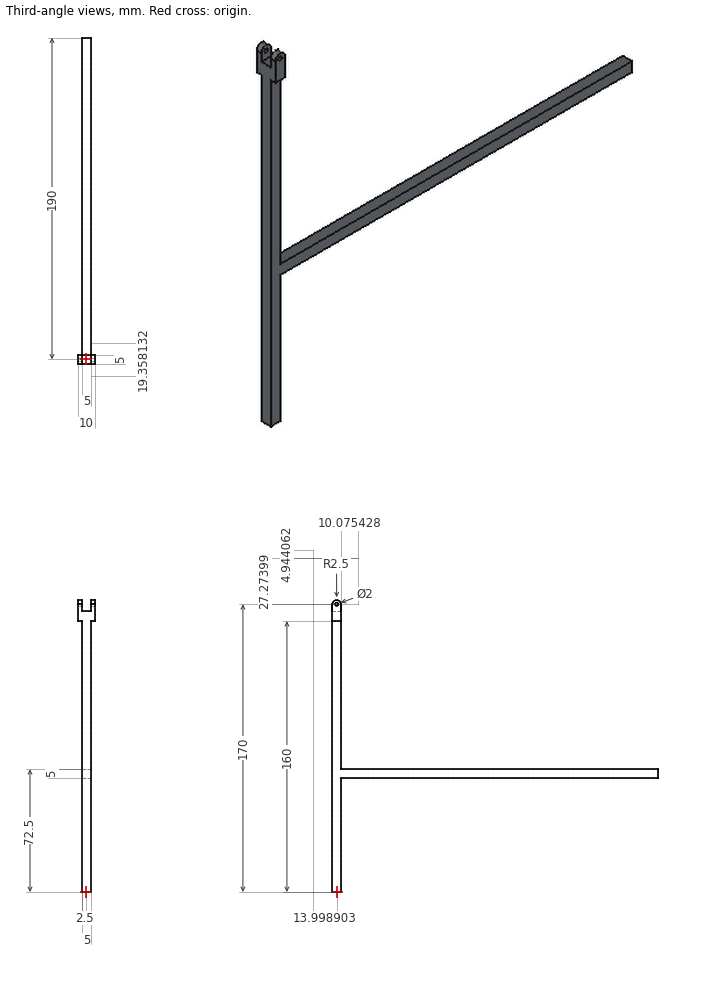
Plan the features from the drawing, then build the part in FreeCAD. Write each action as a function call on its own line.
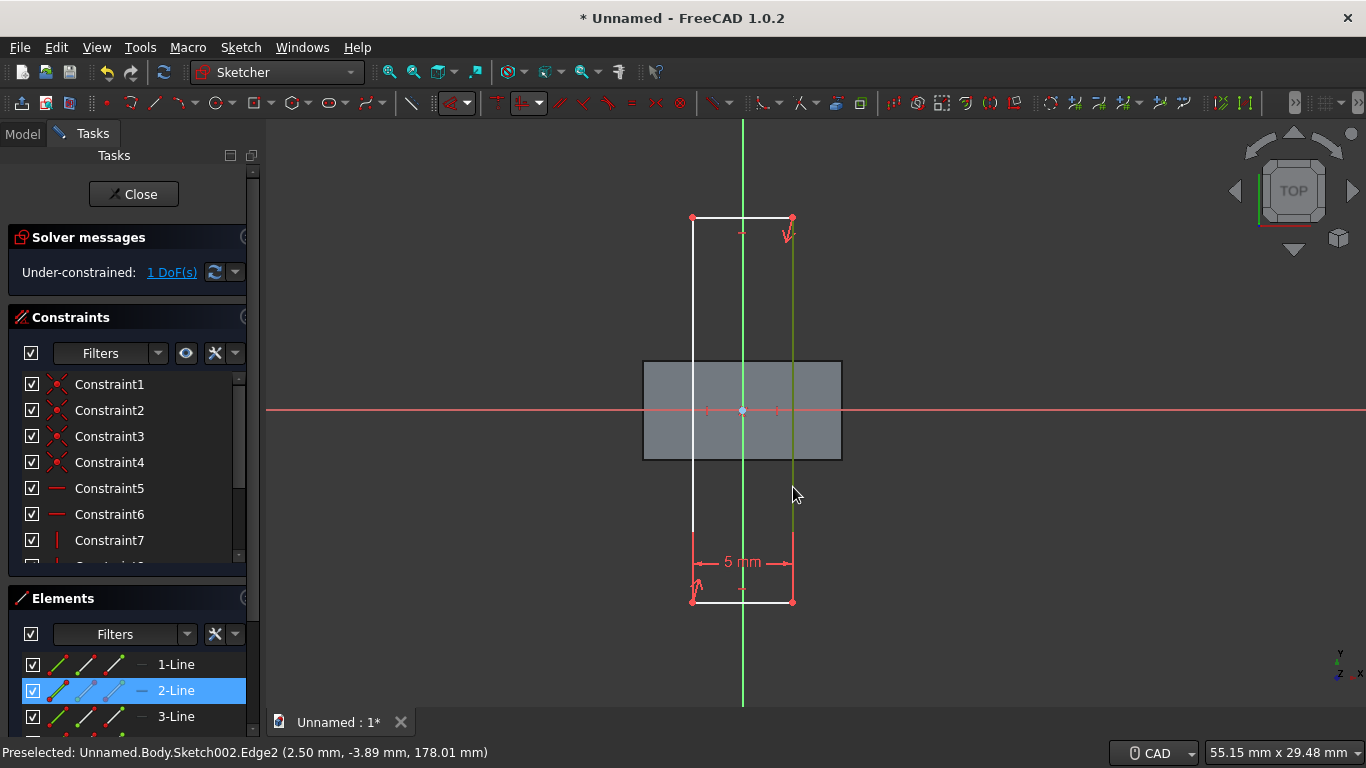
click(470, 104)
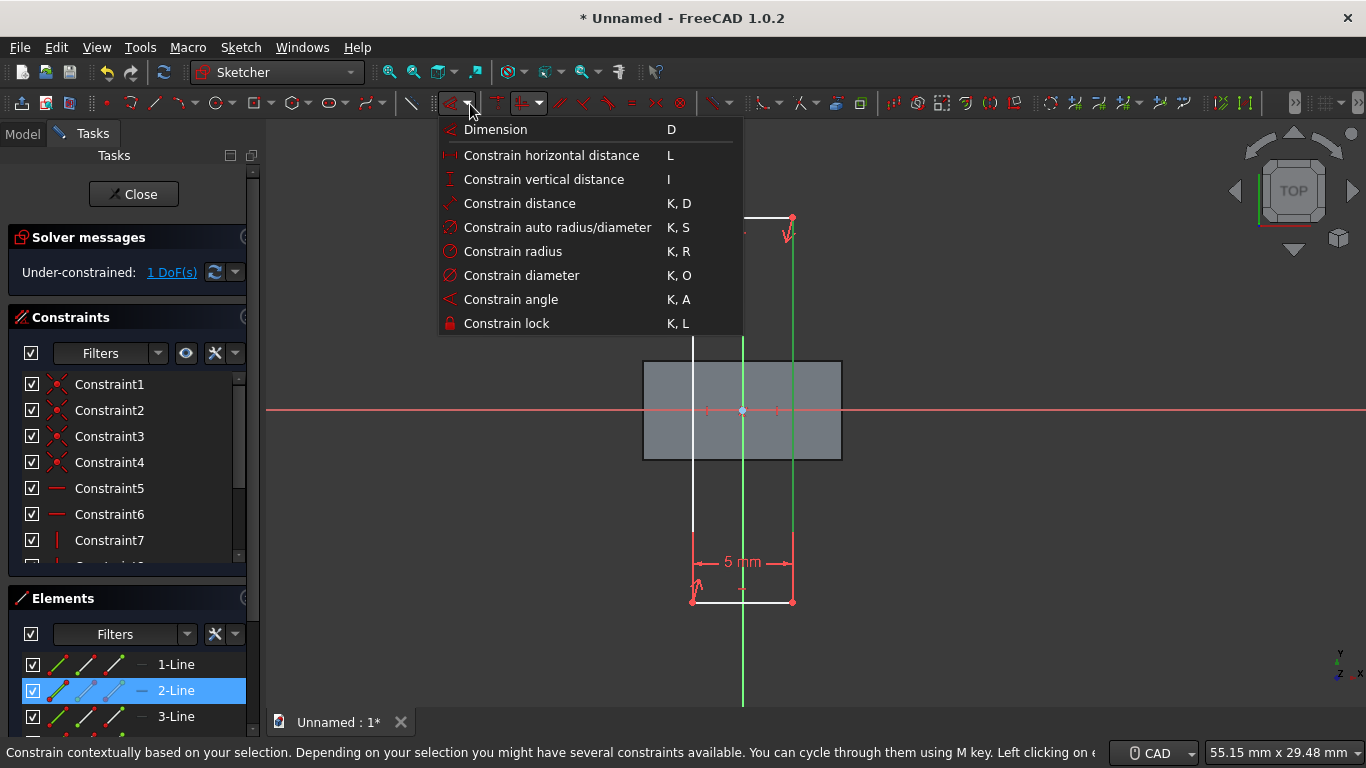
click(591, 179)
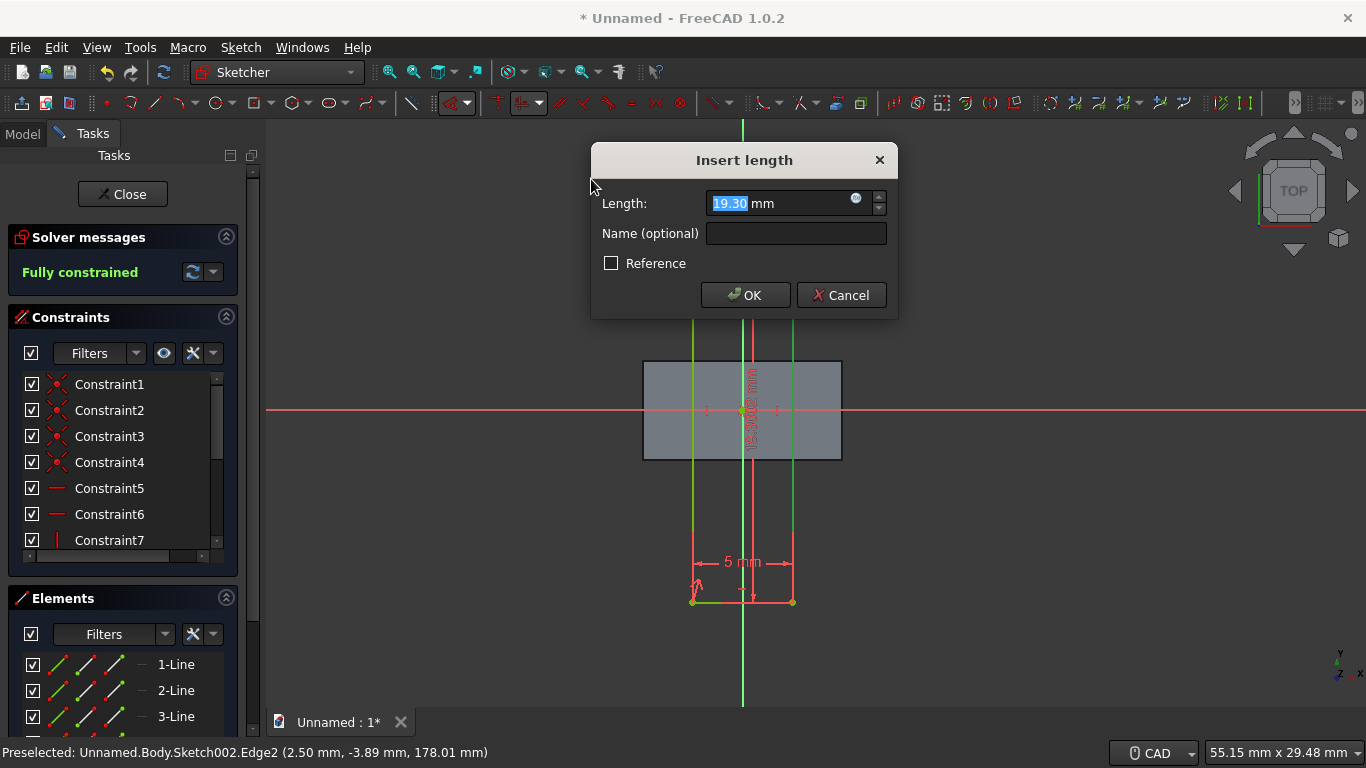
text(19.358132)
key(Return)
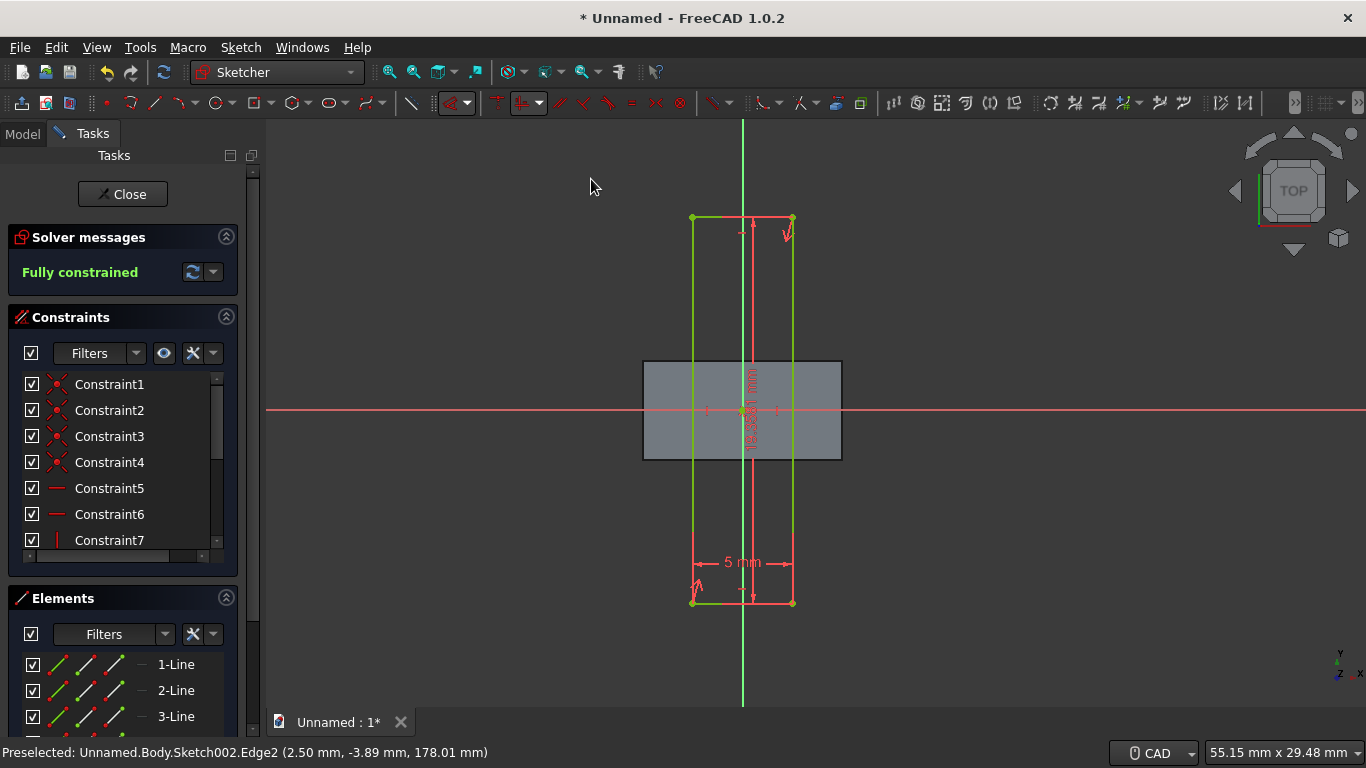
click(123, 194)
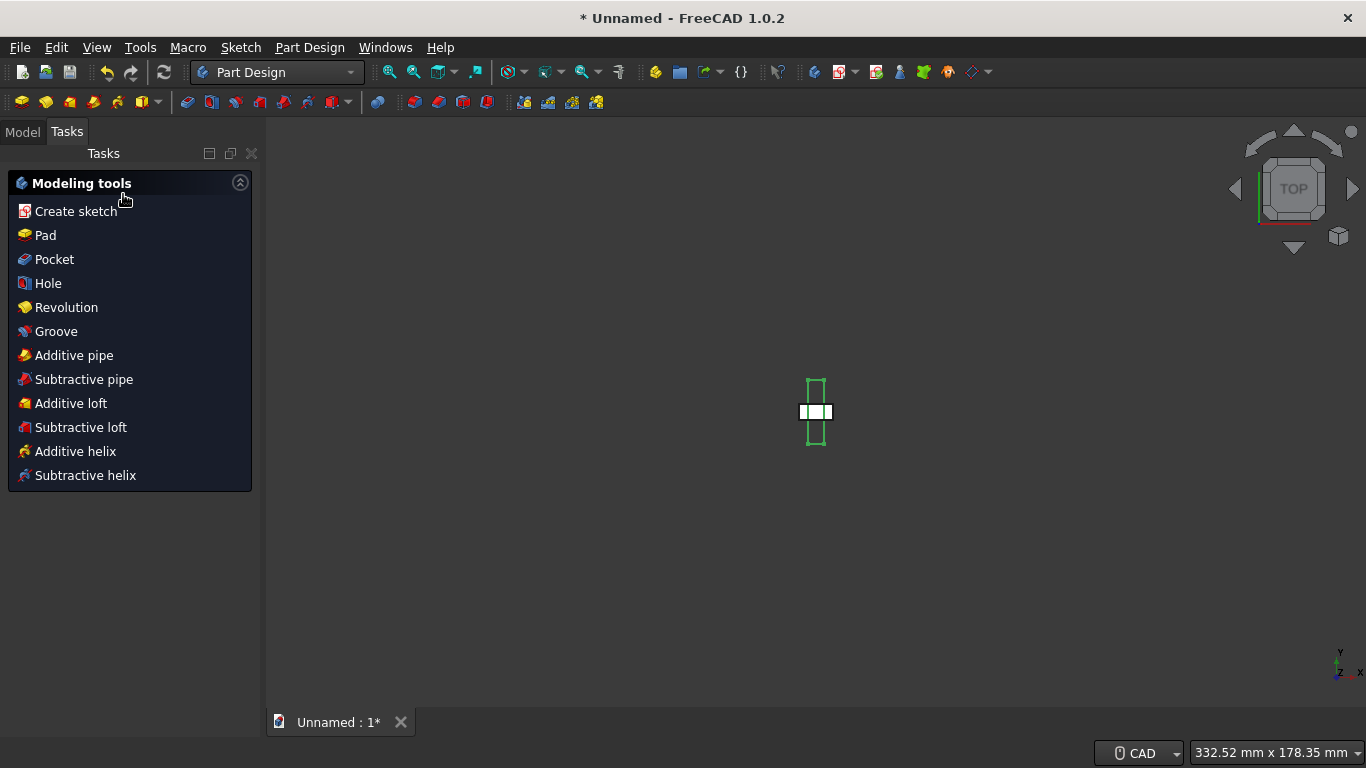
click(188, 102)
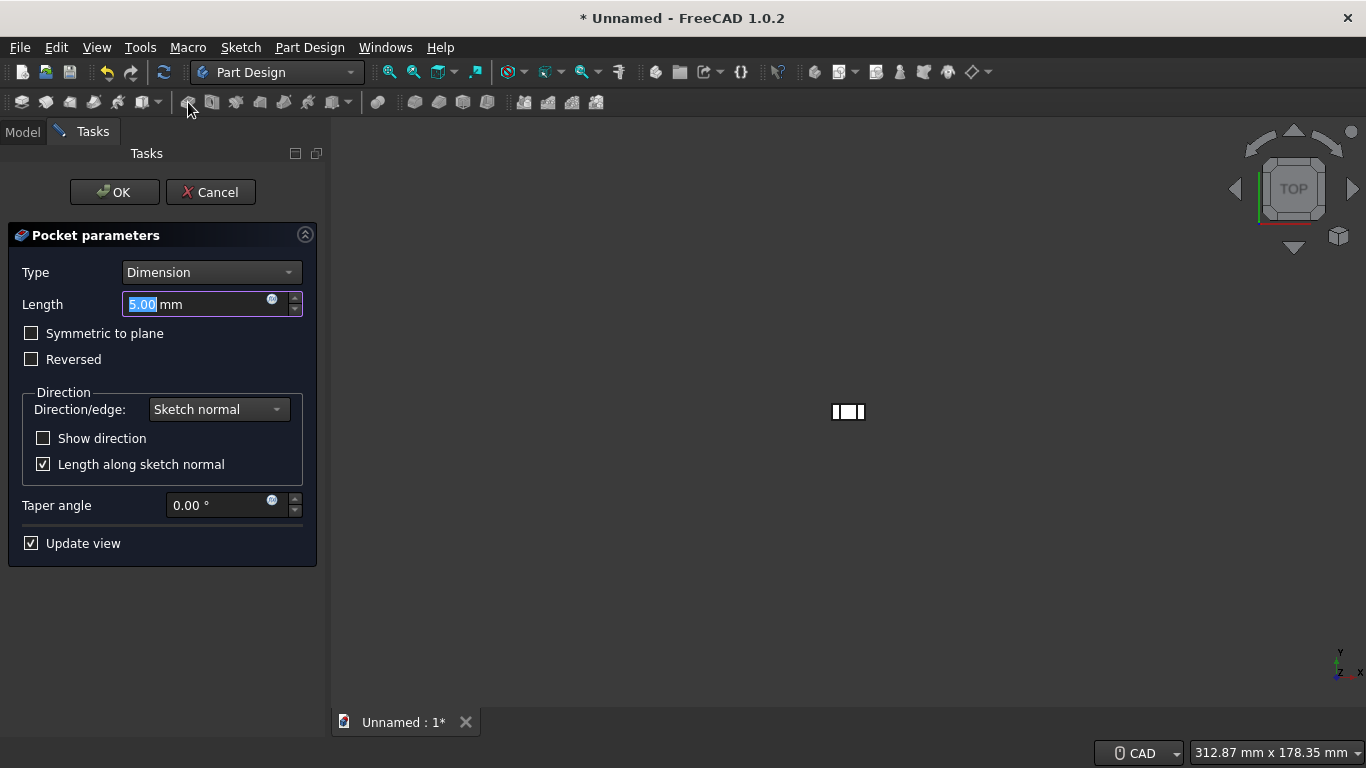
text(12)
key(Tab)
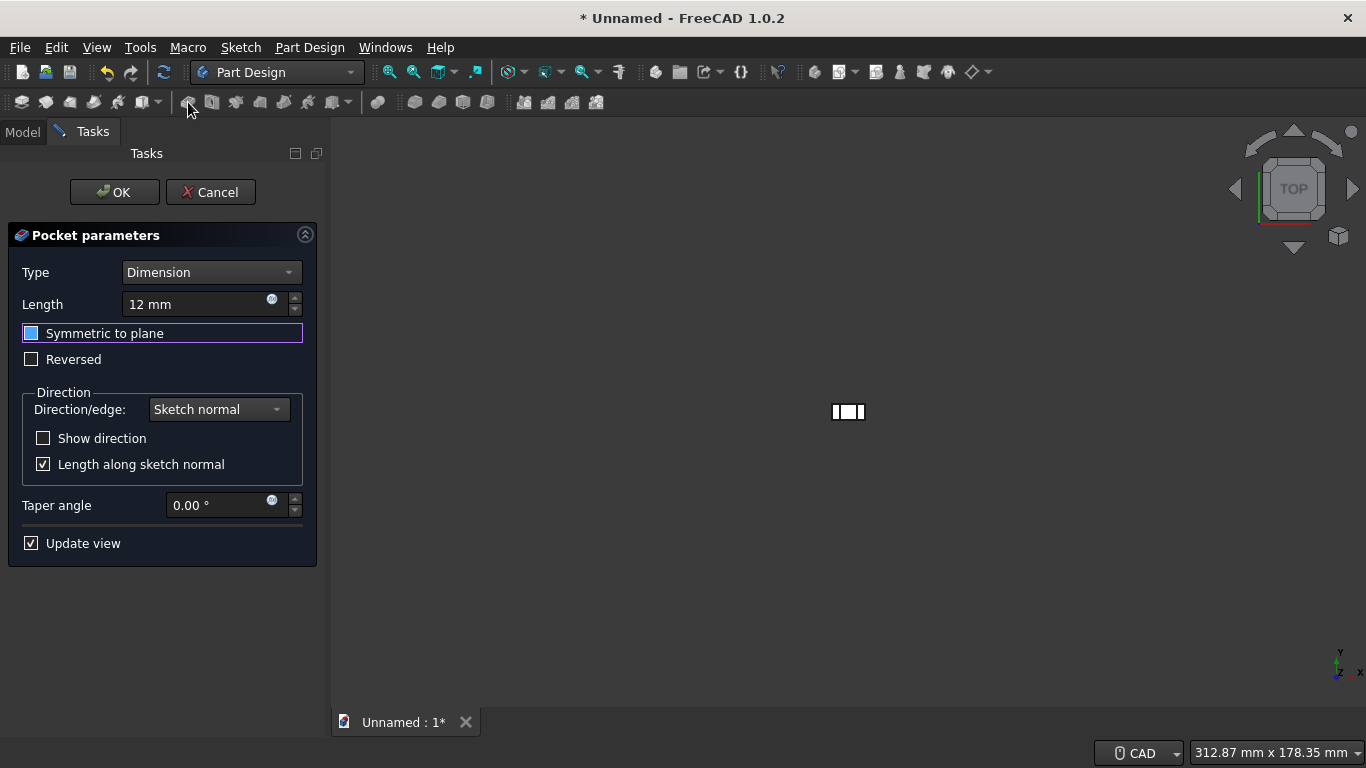
click(115, 192)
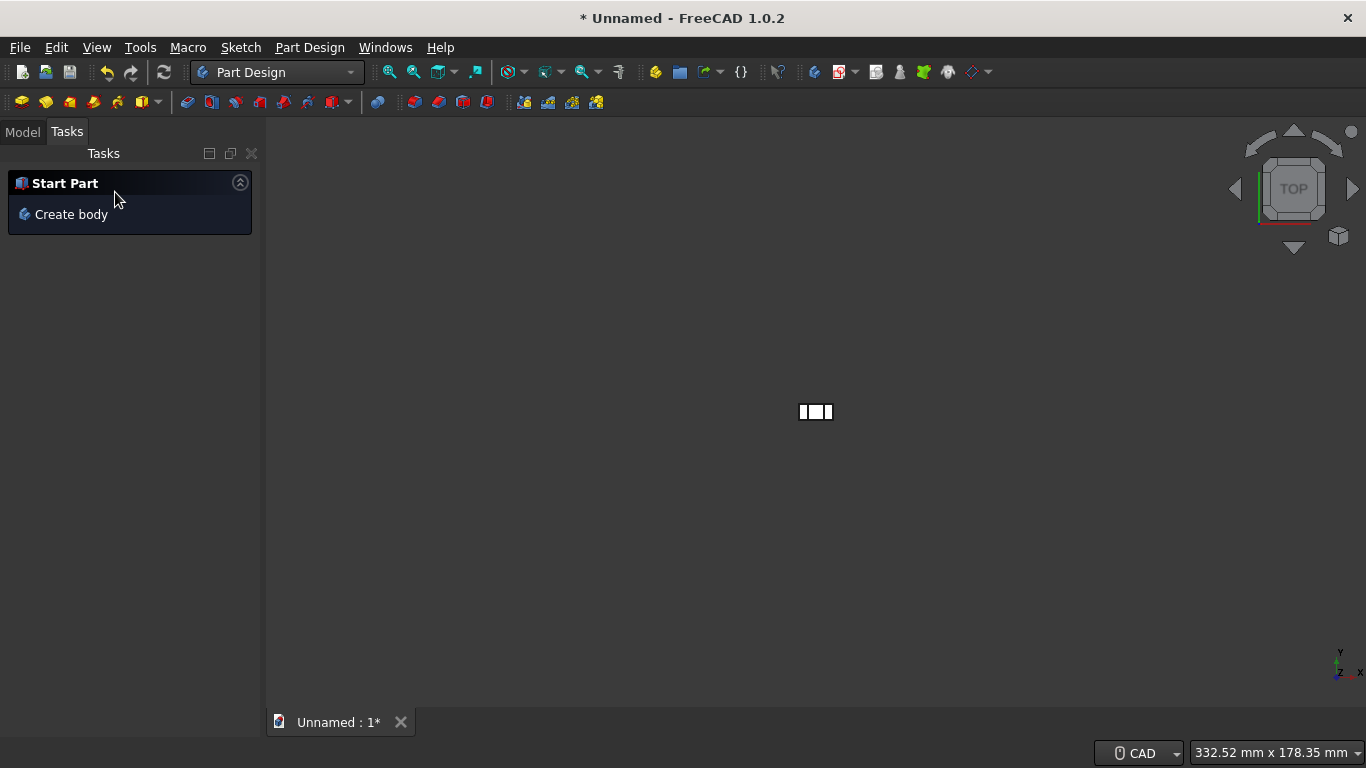
click(390, 72)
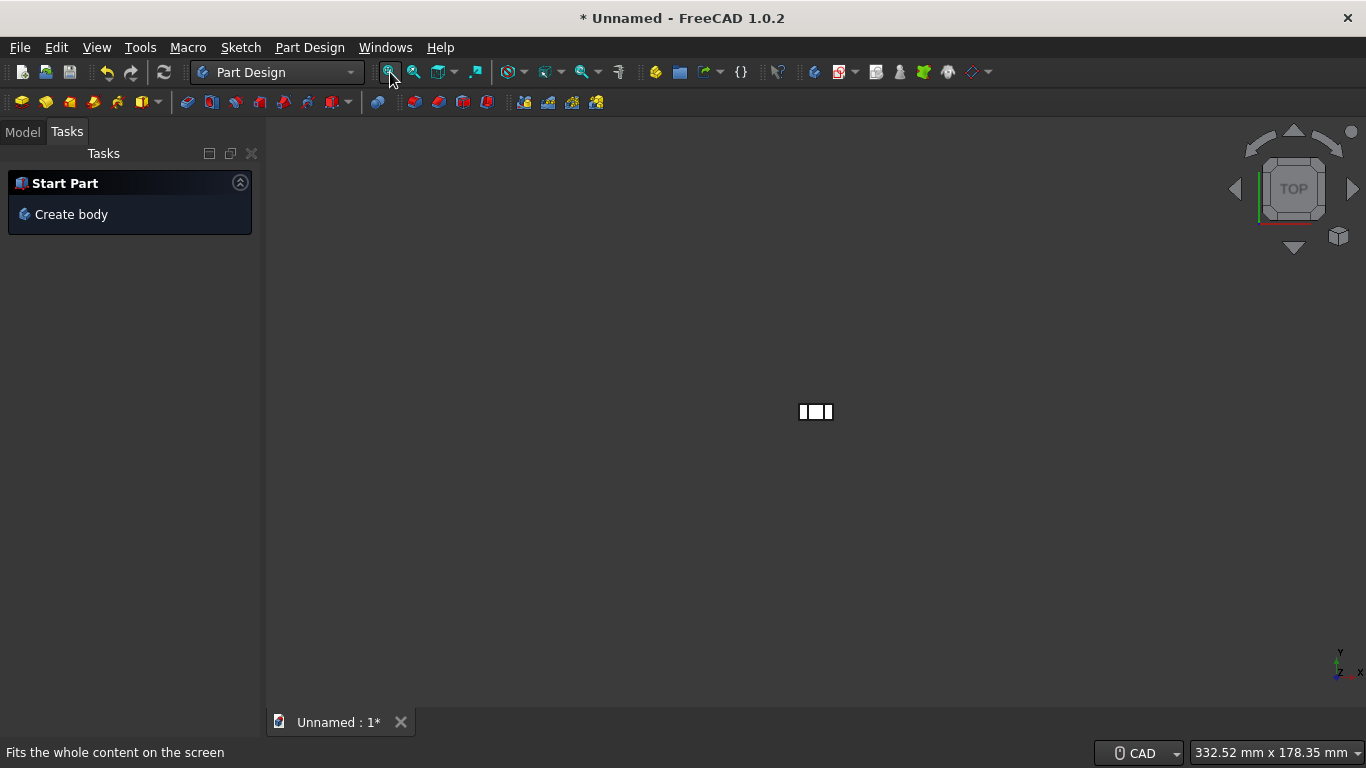
key(0)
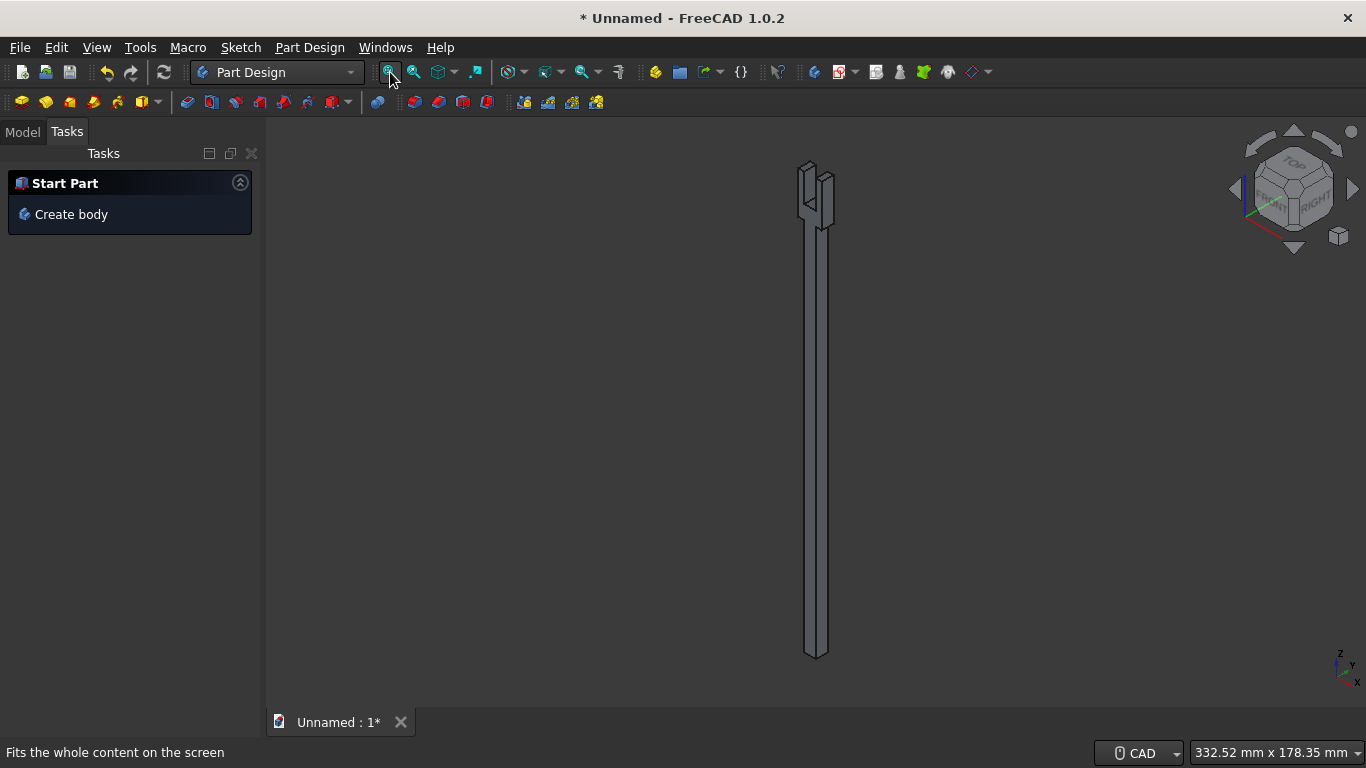
key(3)